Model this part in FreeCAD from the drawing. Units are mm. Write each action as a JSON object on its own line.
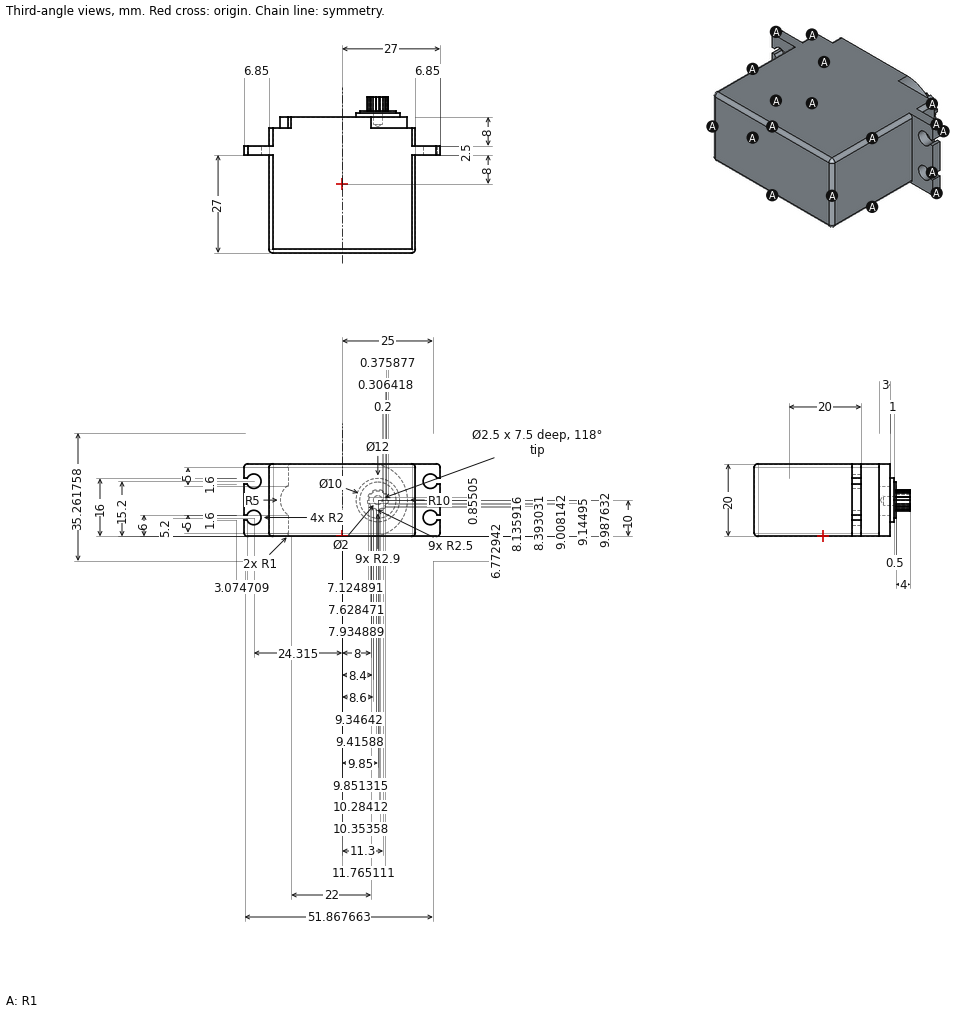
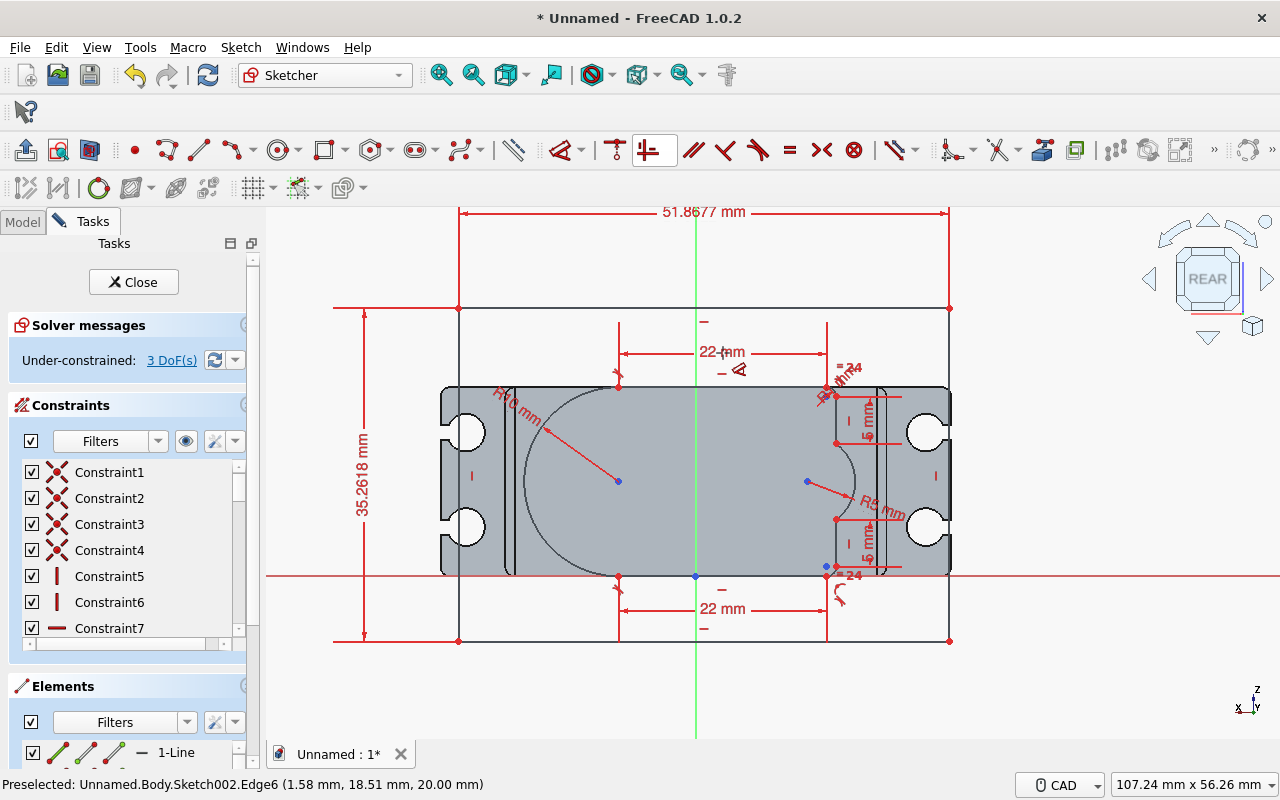
{"action": "left_click", "coordinate": [619, 576]}
{"action": "left_click", "coordinate": [640, 610]}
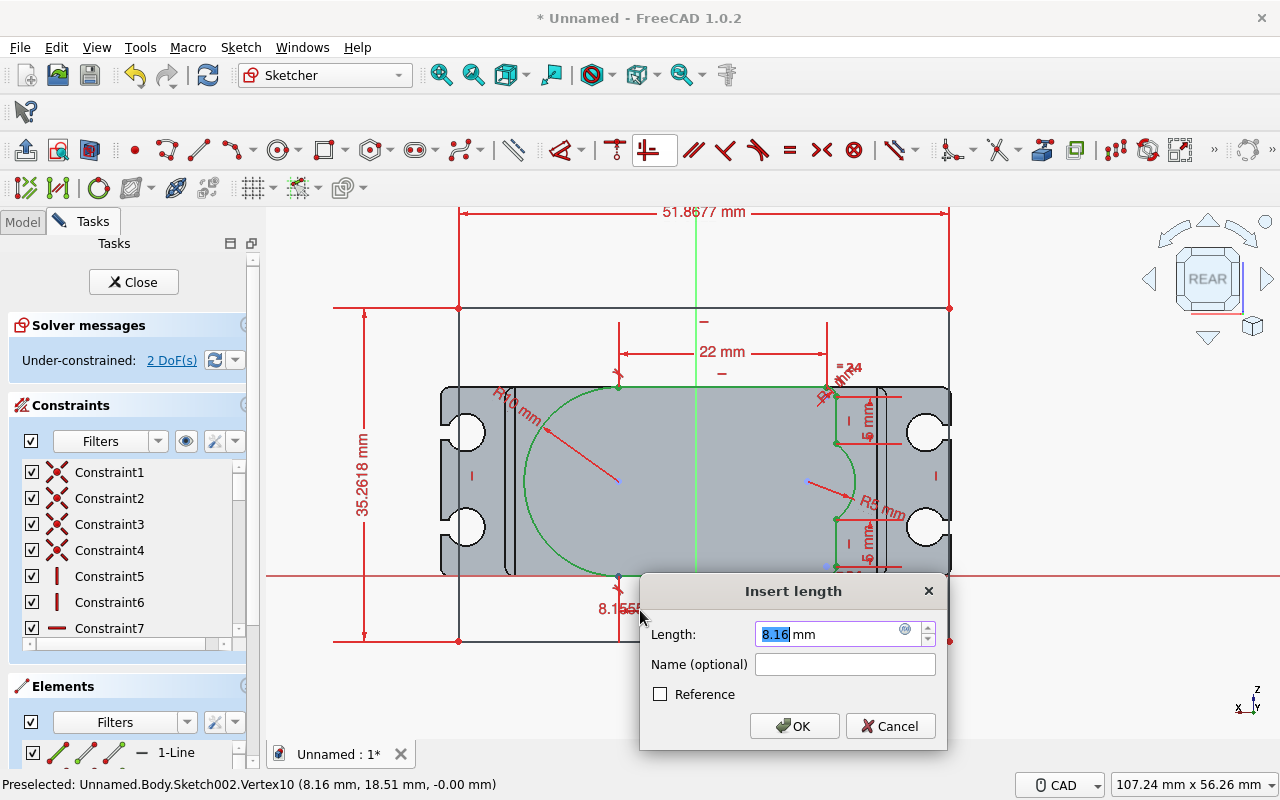
{"action": "type", "text": "8"}
{"action": "key", "text": "Return"}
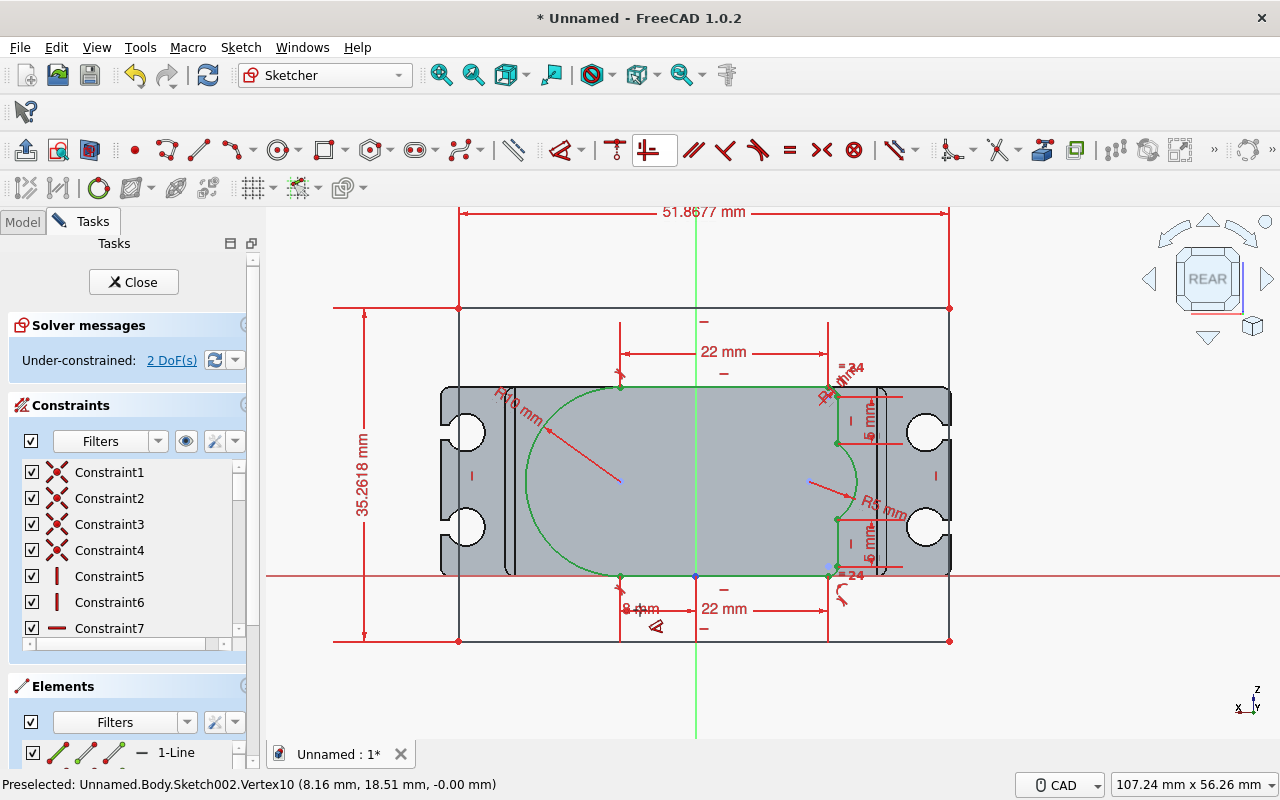
{"action": "left_click", "coordinate": [459, 308]}
{"action": "left_click", "coordinate": [577, 274]}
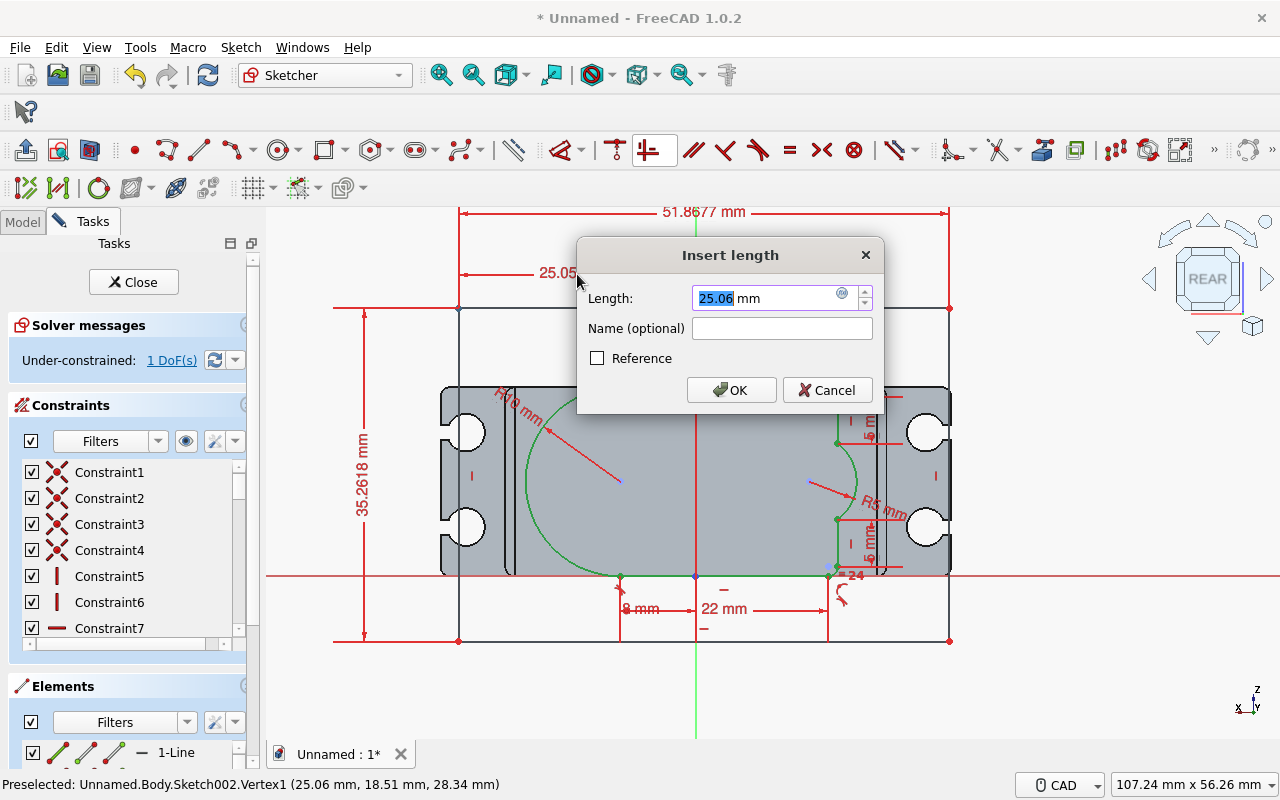
{"action": "type", "text": "25"}
{"action": "key", "text": "Return"}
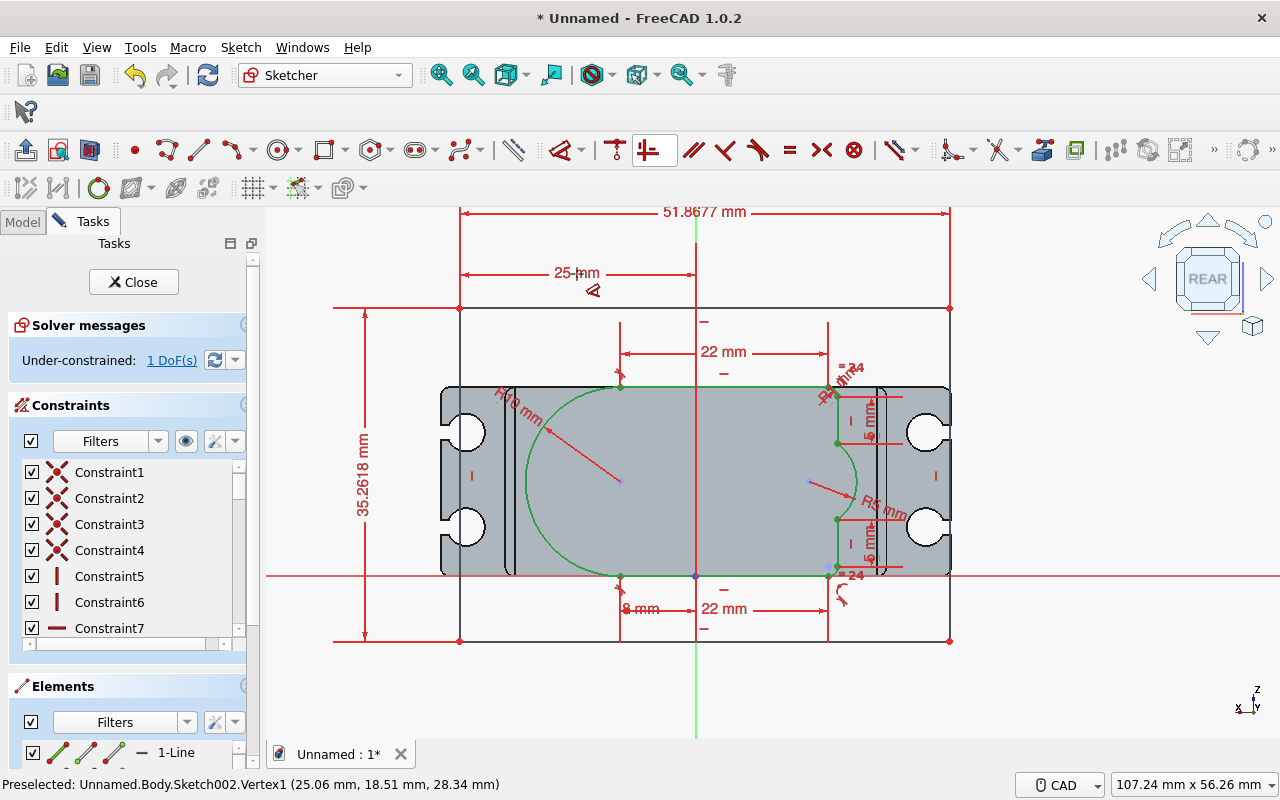
{"action": "left_click", "coordinate": [460, 642]}
{"action": "left_click", "coordinate": [426, 609]}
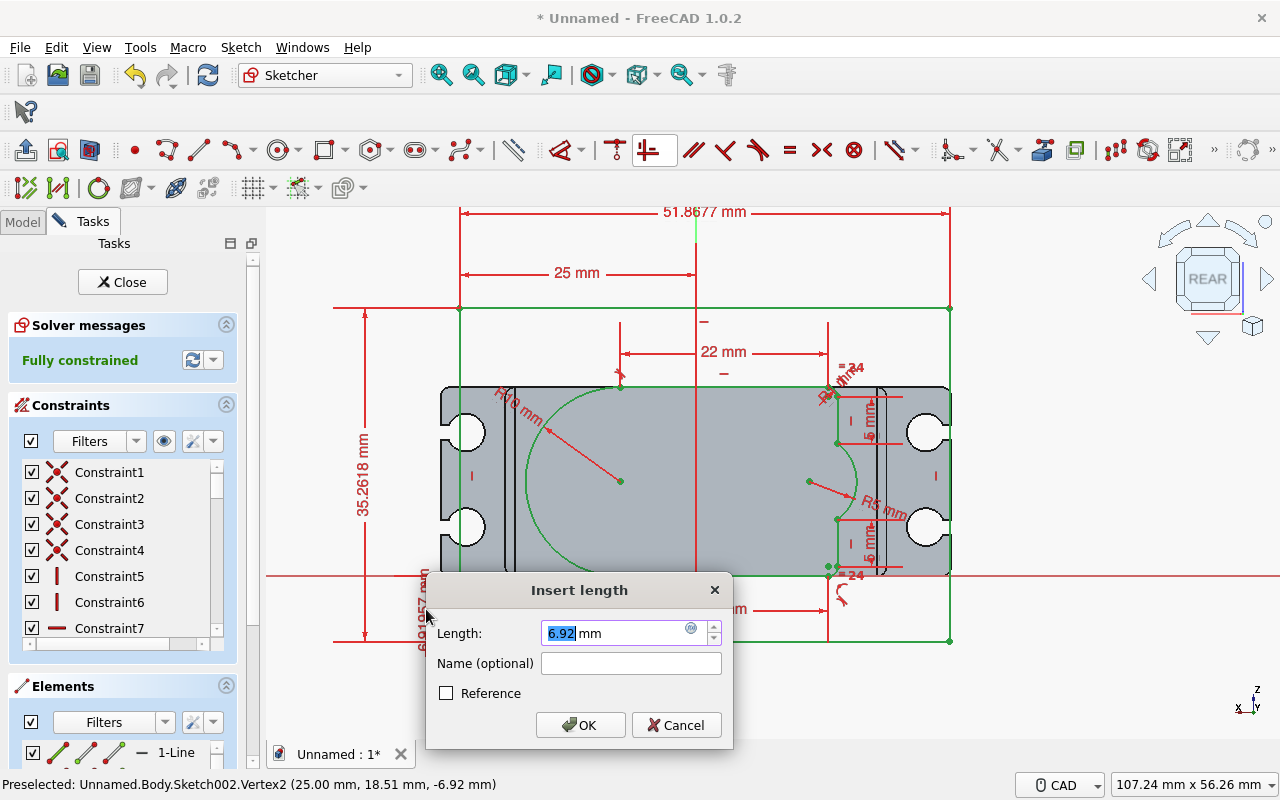
{"action": "type", "text": "6.772942"}
{"action": "key", "text": "Return"}
{"action": "key", "text": "Escape"}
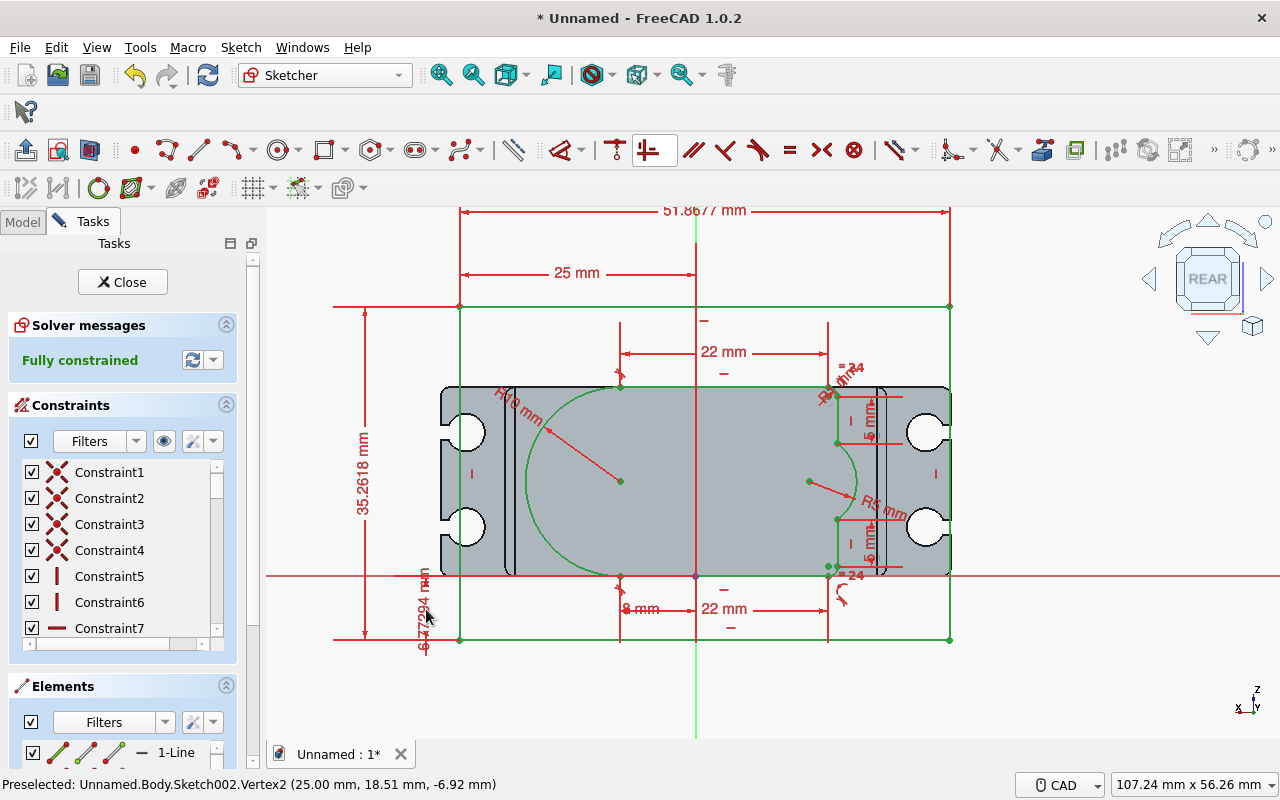
{"action": "left_click", "coordinate": [123, 282]}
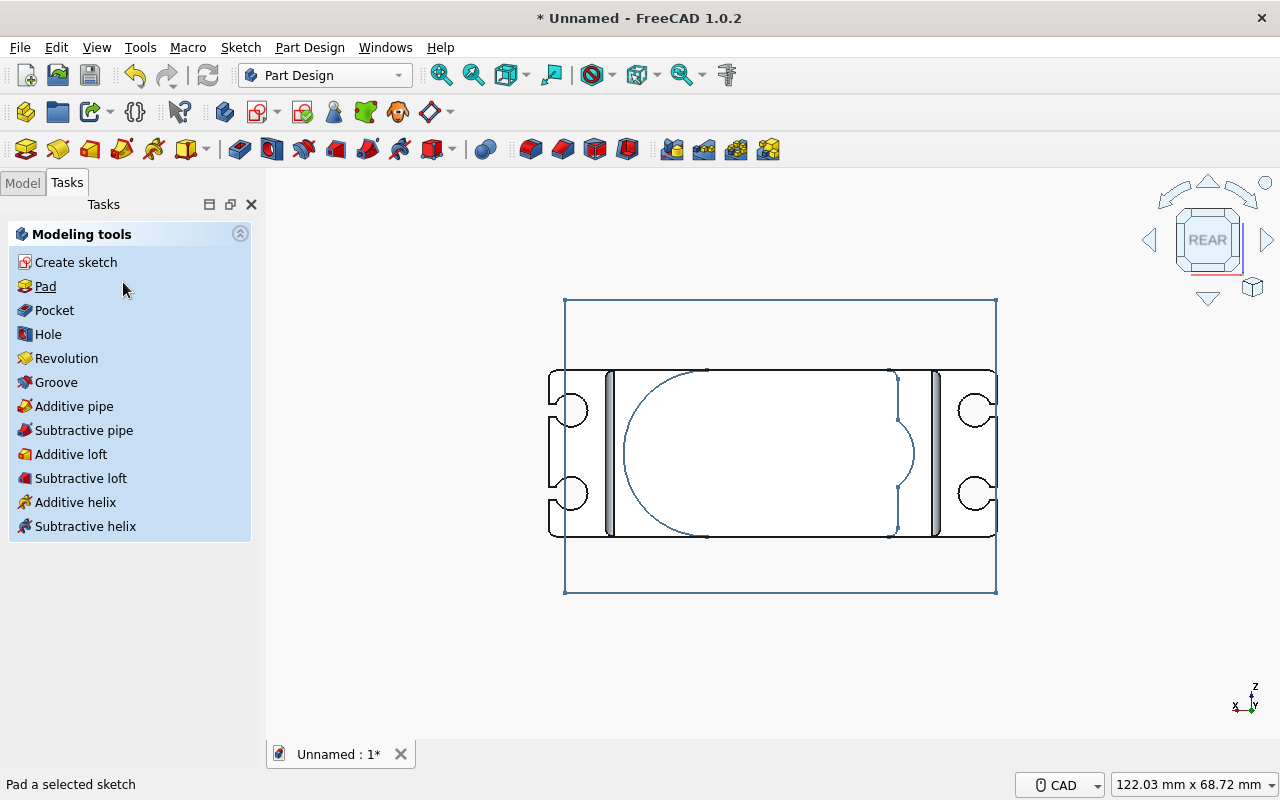
{"action": "left_click", "coordinate": [240, 150]}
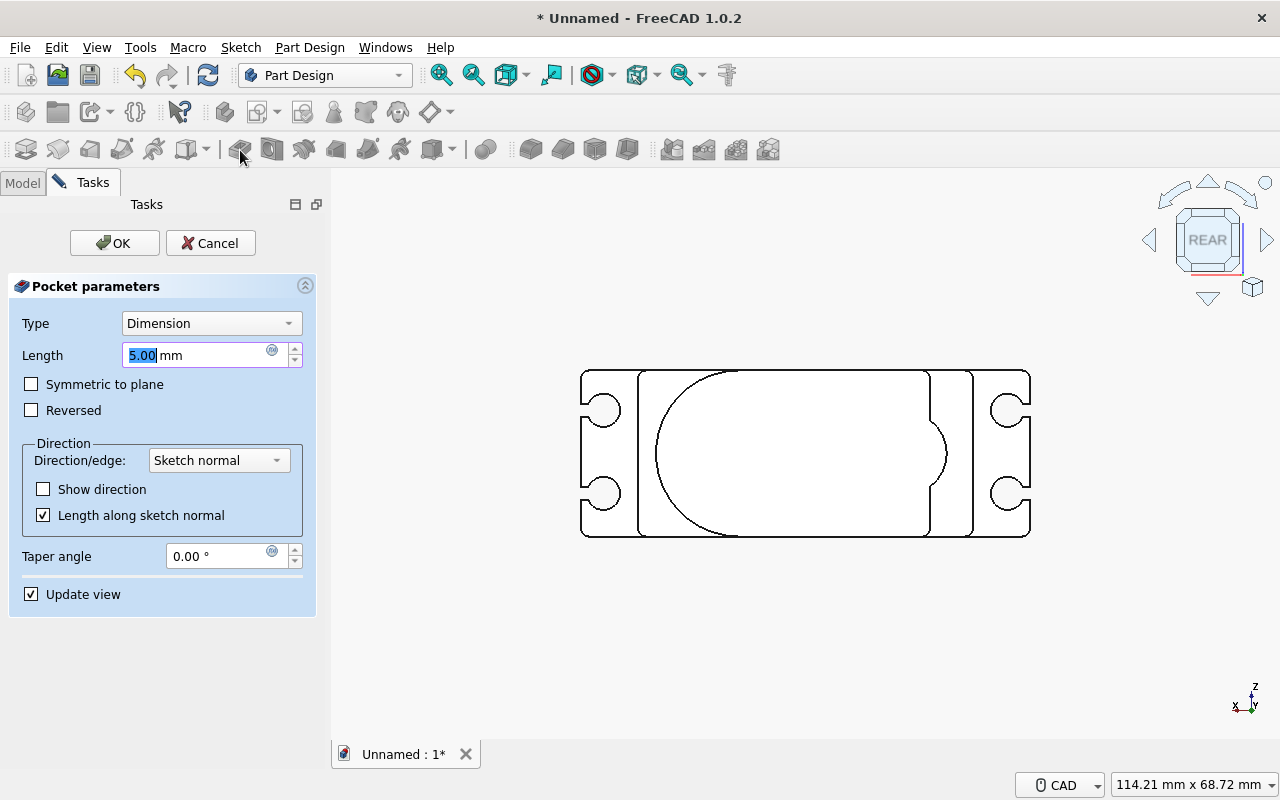
{"action": "type", "text": "3"}
{"action": "key", "text": "Tab"}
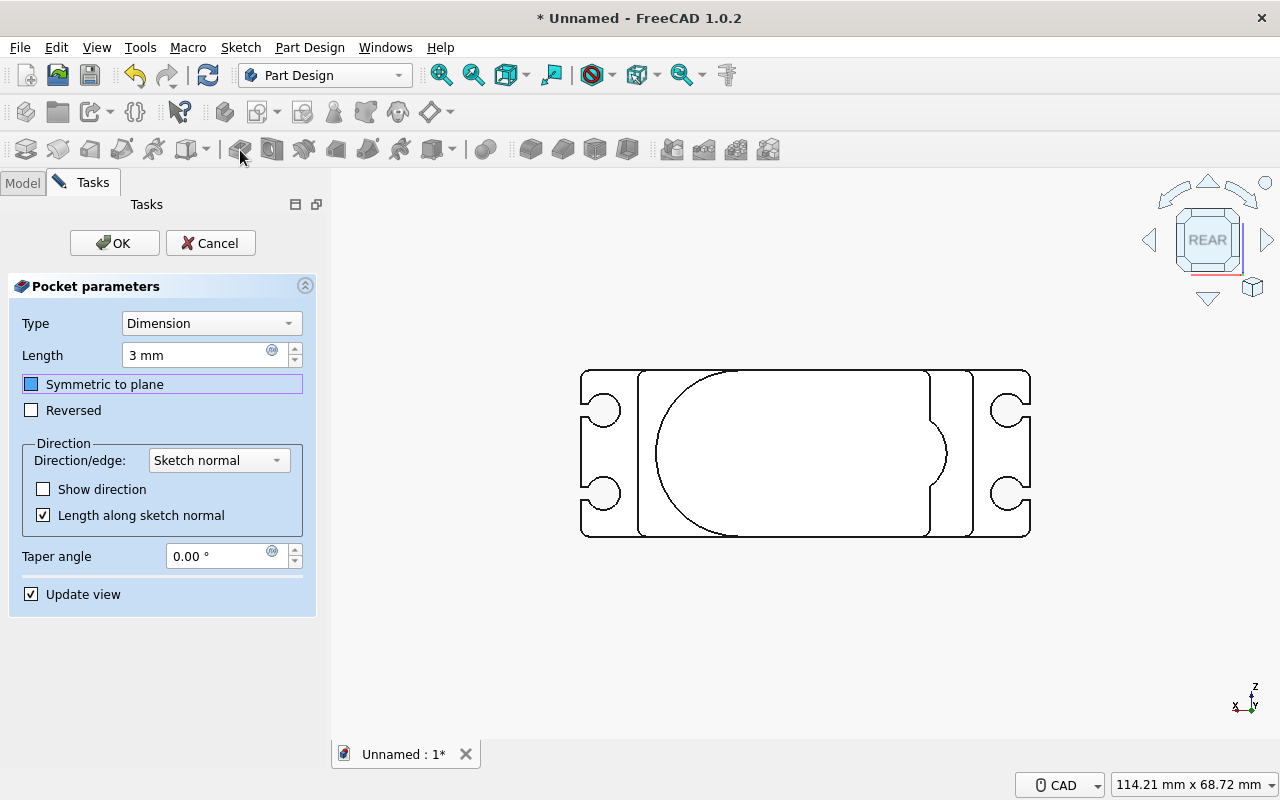
{"action": "left_click", "coordinate": [115, 243]}